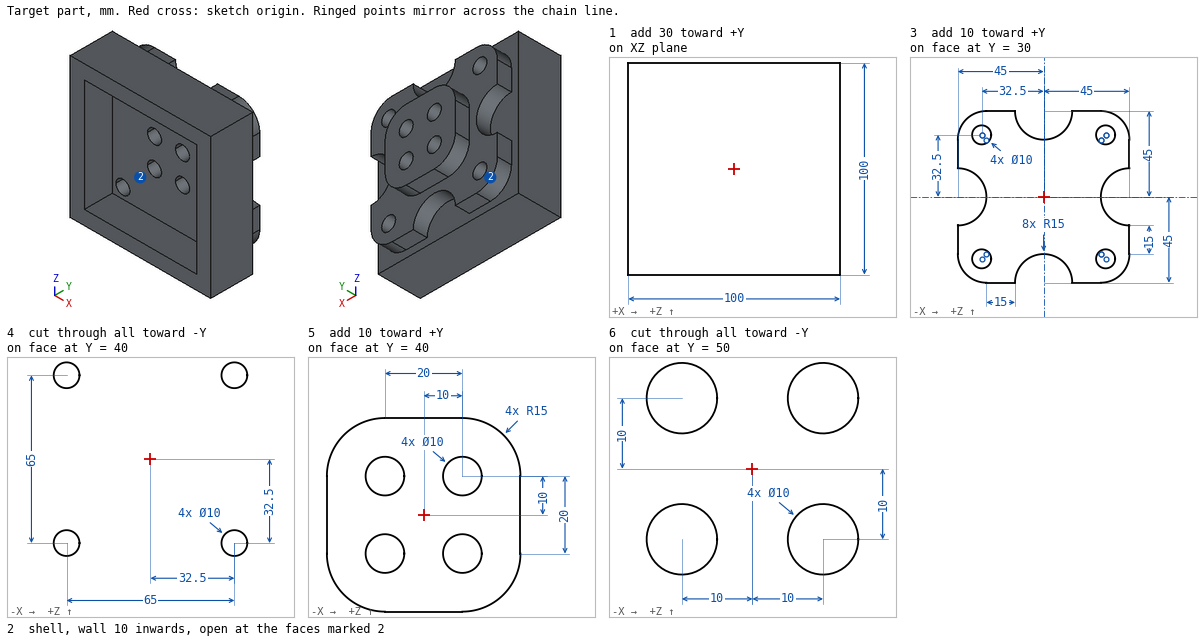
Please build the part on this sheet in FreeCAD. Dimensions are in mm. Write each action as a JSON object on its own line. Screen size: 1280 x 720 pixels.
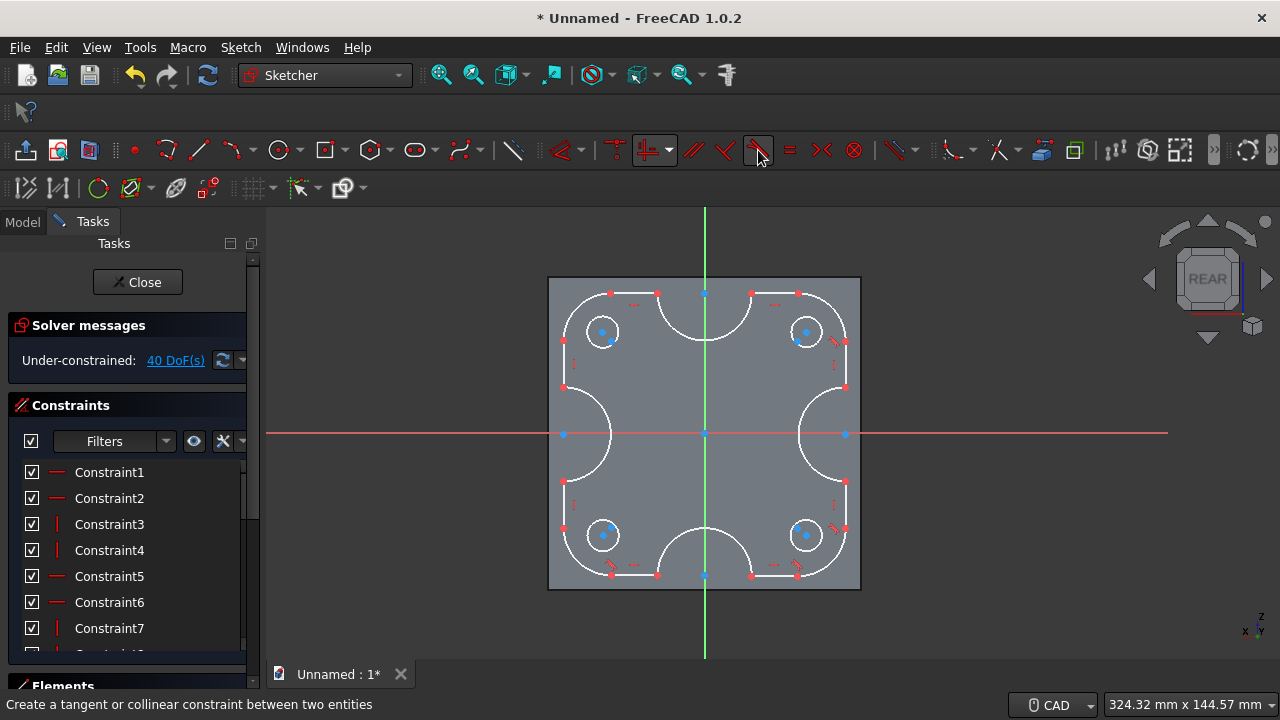
{"action": "left_click", "coordinate": [785, 293]}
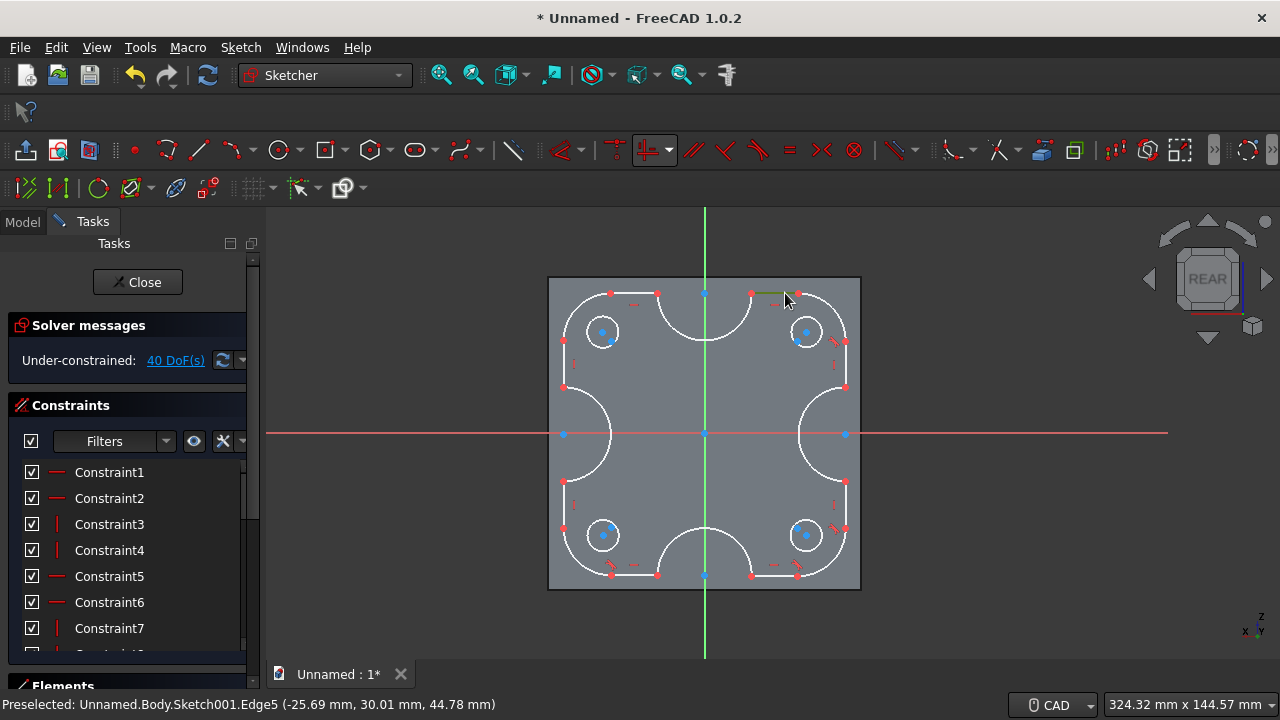
{"action": "left_click", "coordinate": [841, 320]}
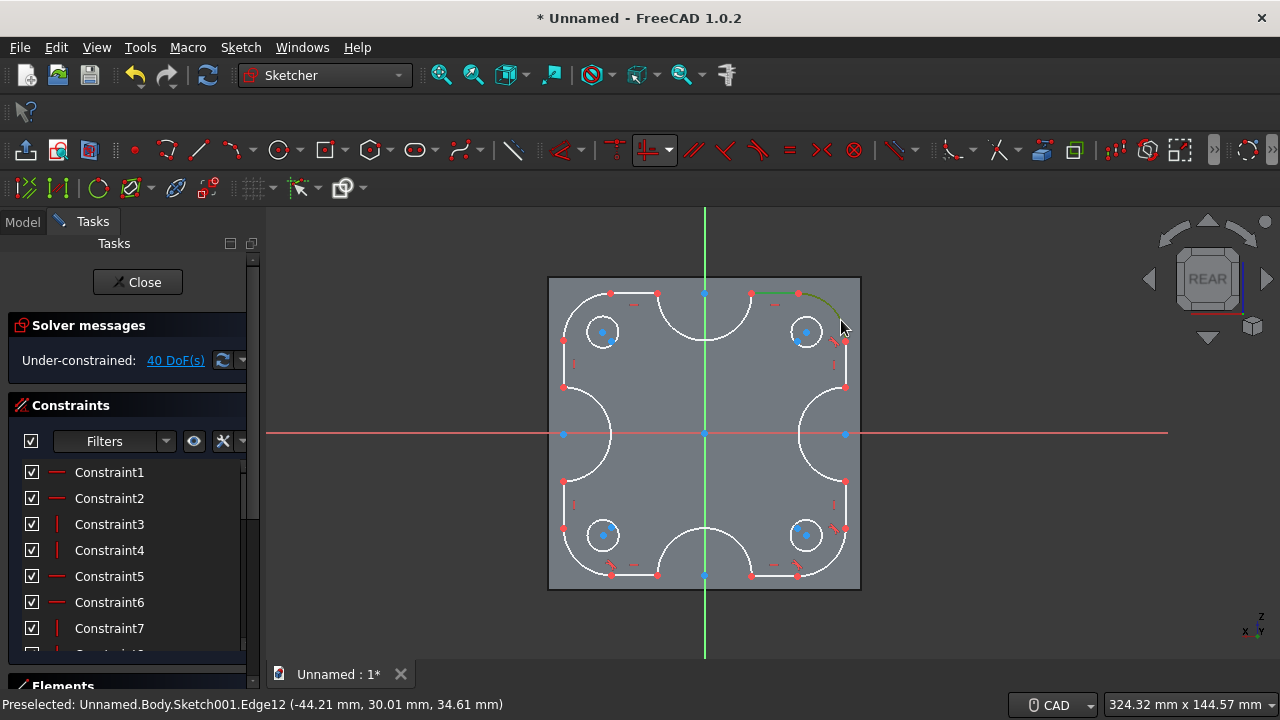
{"action": "left_click", "coordinate": [758, 150]}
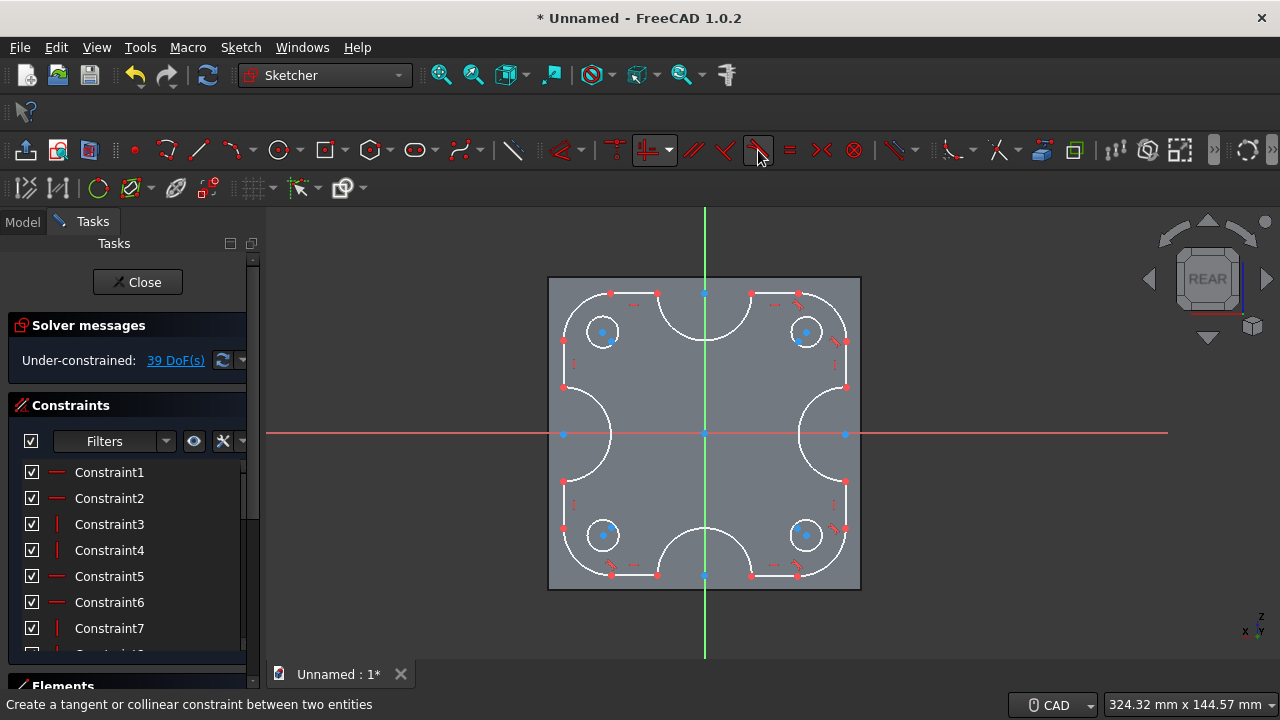
{"action": "left_click", "coordinate": [644, 293]}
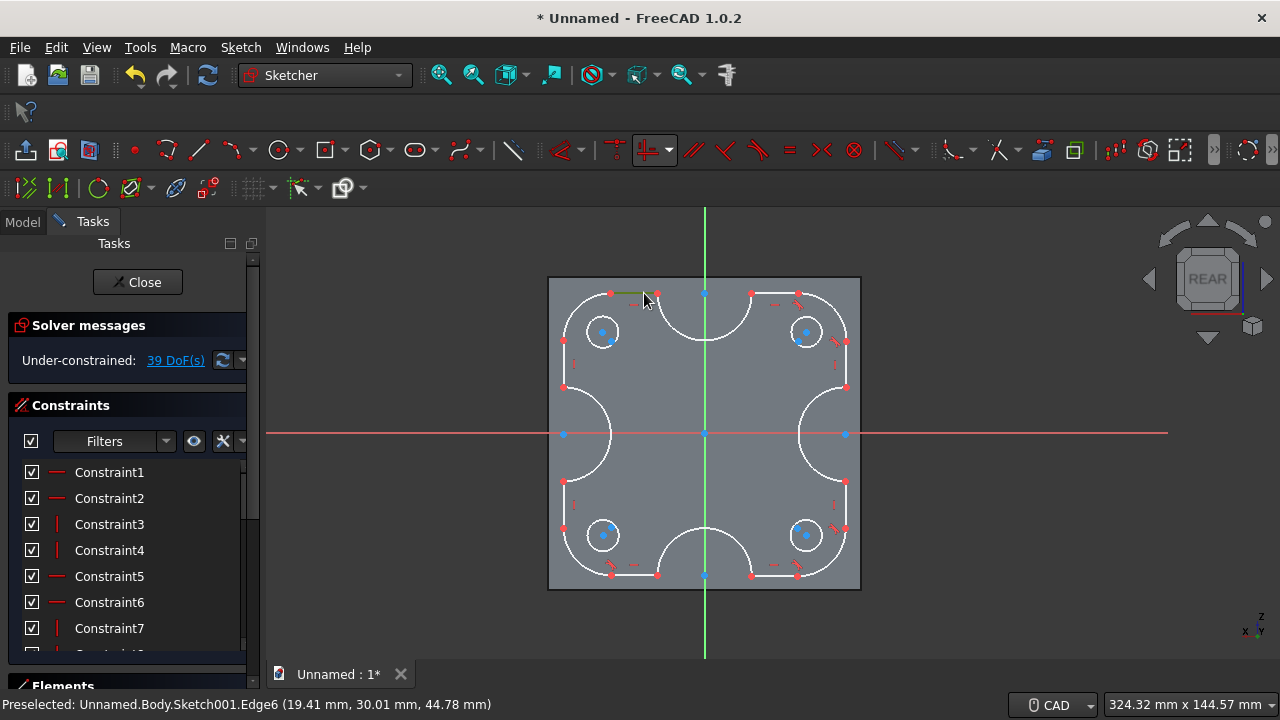
{"action": "left_click", "coordinate": [590, 299]}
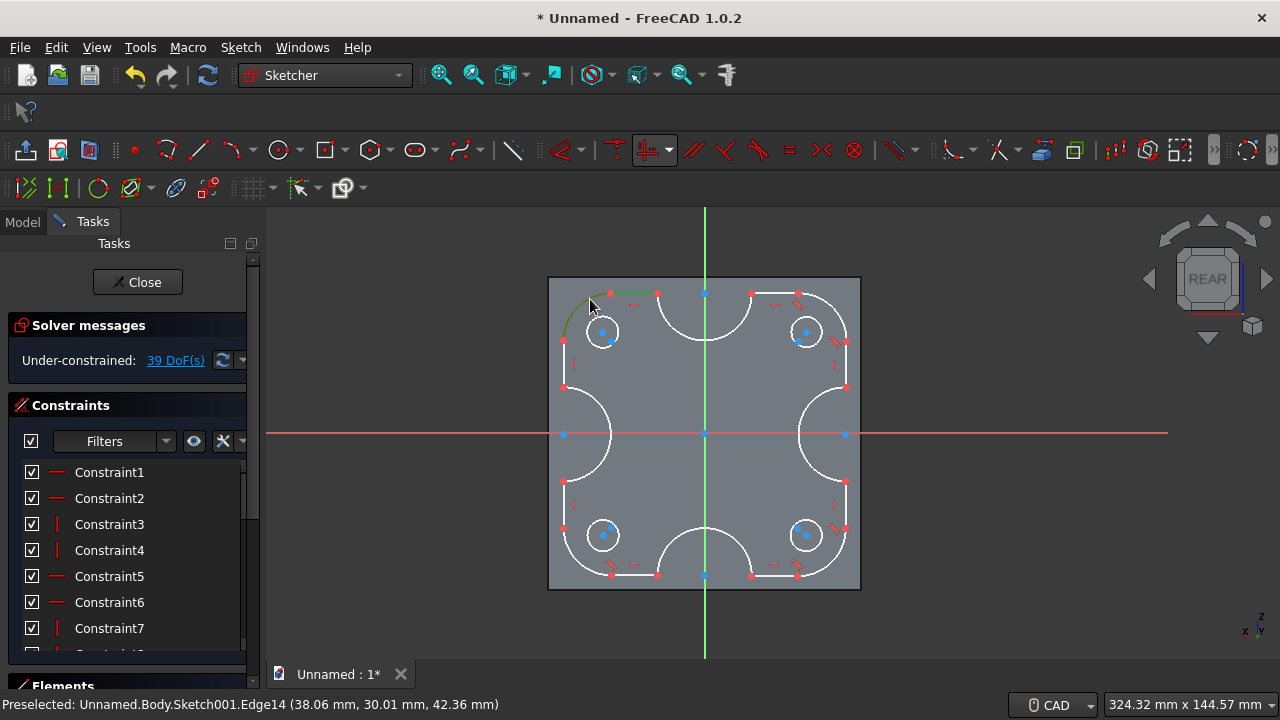
{"action": "left_click", "coordinate": [758, 150]}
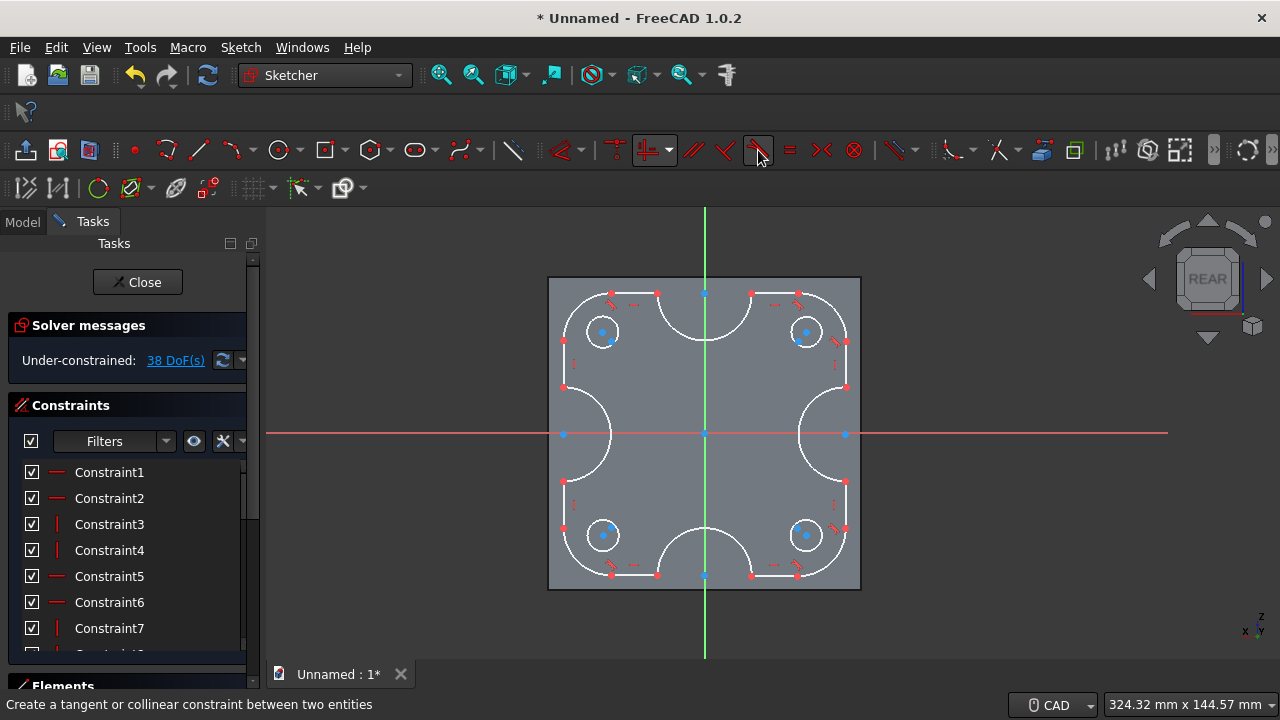
{"action": "left_click", "coordinate": [564, 354]}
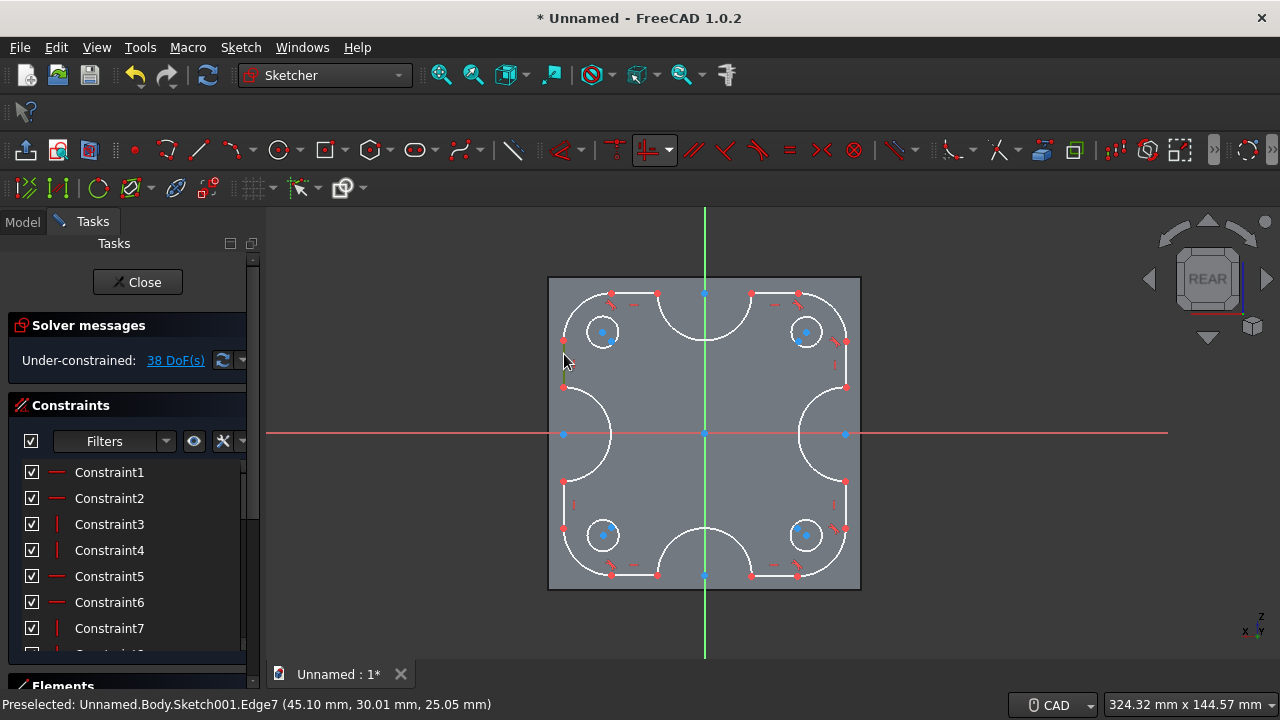
{"action": "left_click", "coordinate": [590, 298]}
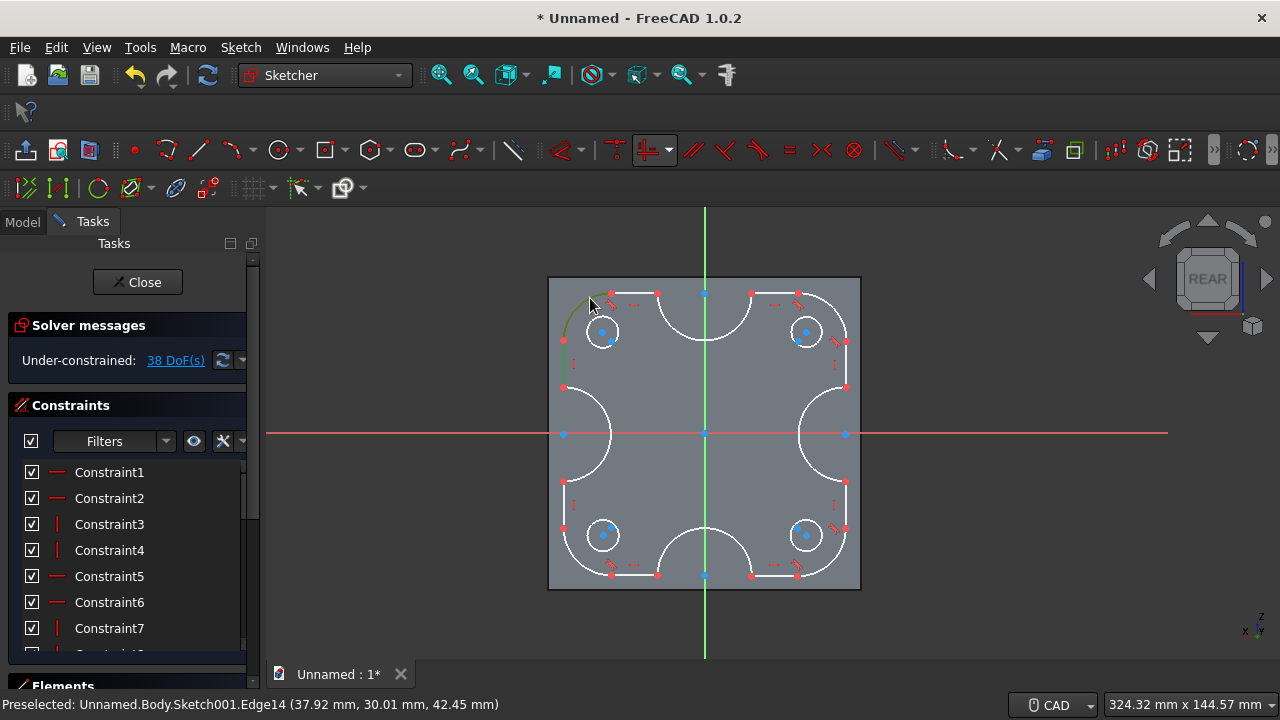
{"action": "left_click", "coordinate": [758, 150]}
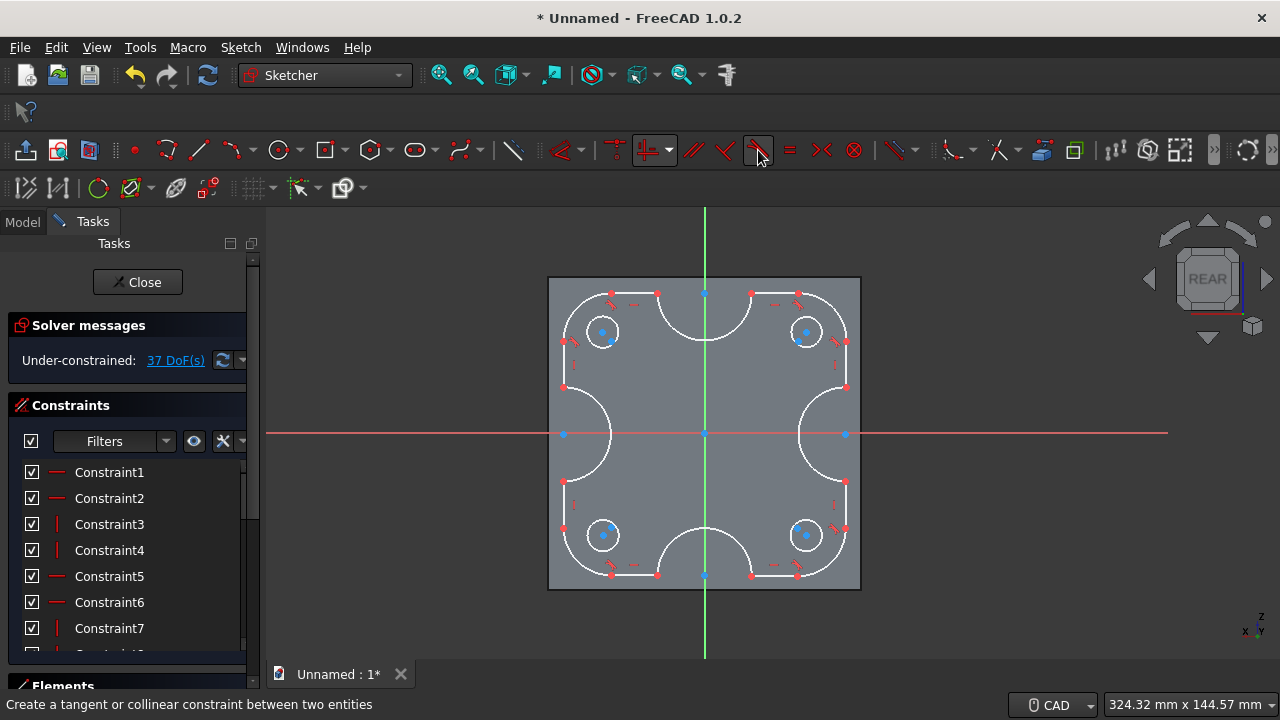
{"action": "left_click", "coordinate": [564, 495]}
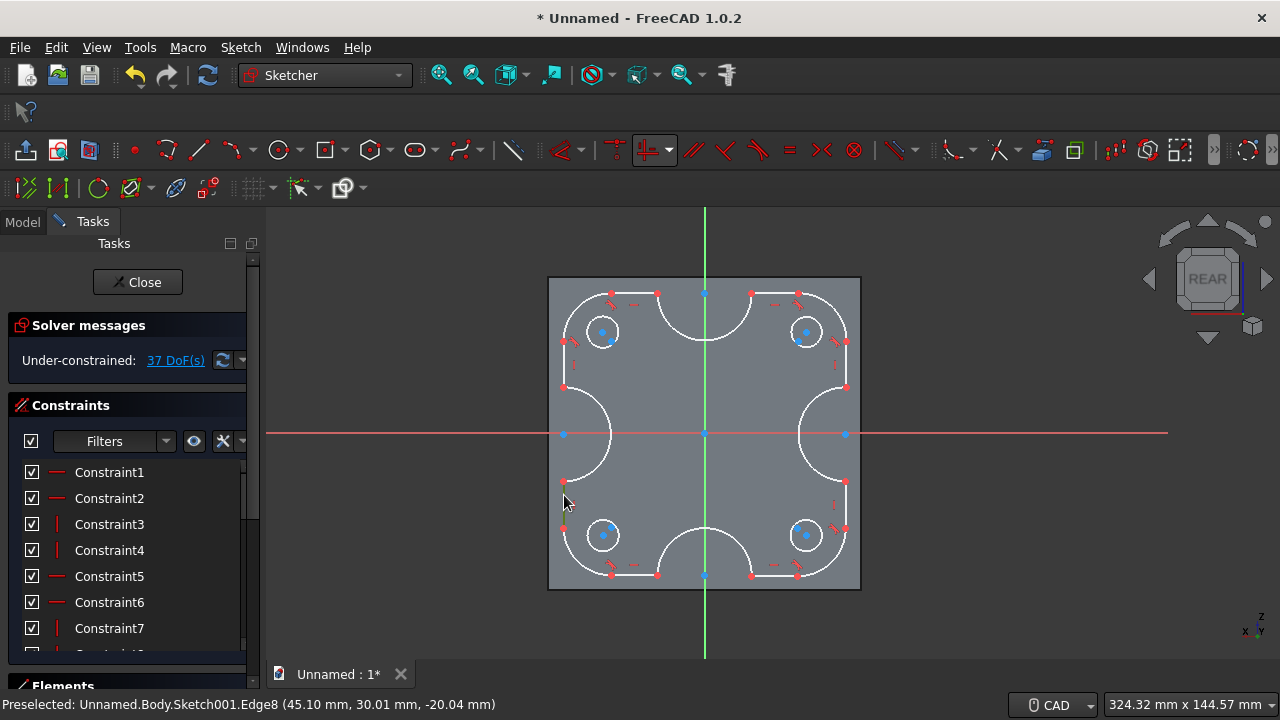
{"action": "left_click", "coordinate": [569, 550]}